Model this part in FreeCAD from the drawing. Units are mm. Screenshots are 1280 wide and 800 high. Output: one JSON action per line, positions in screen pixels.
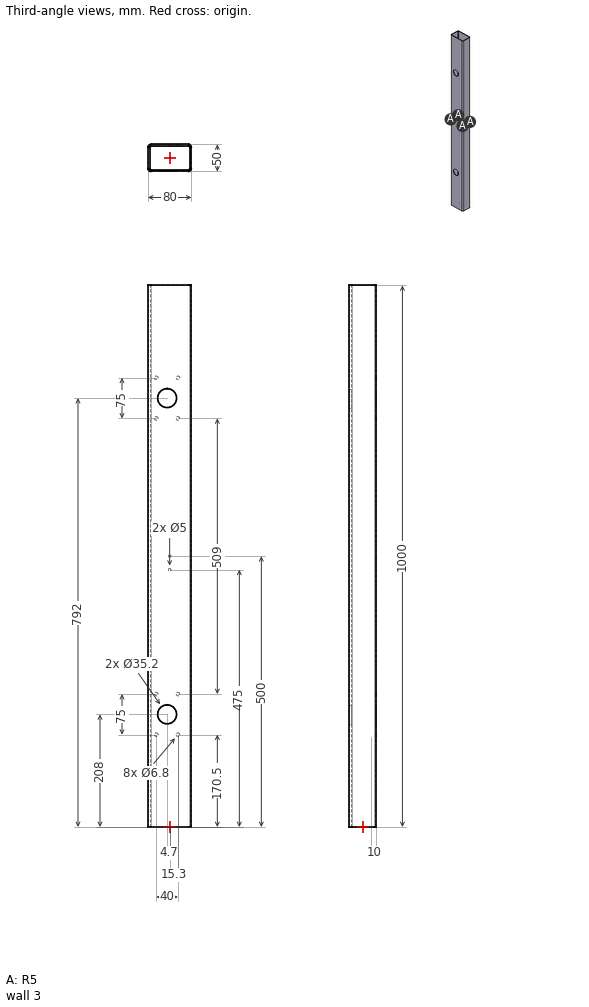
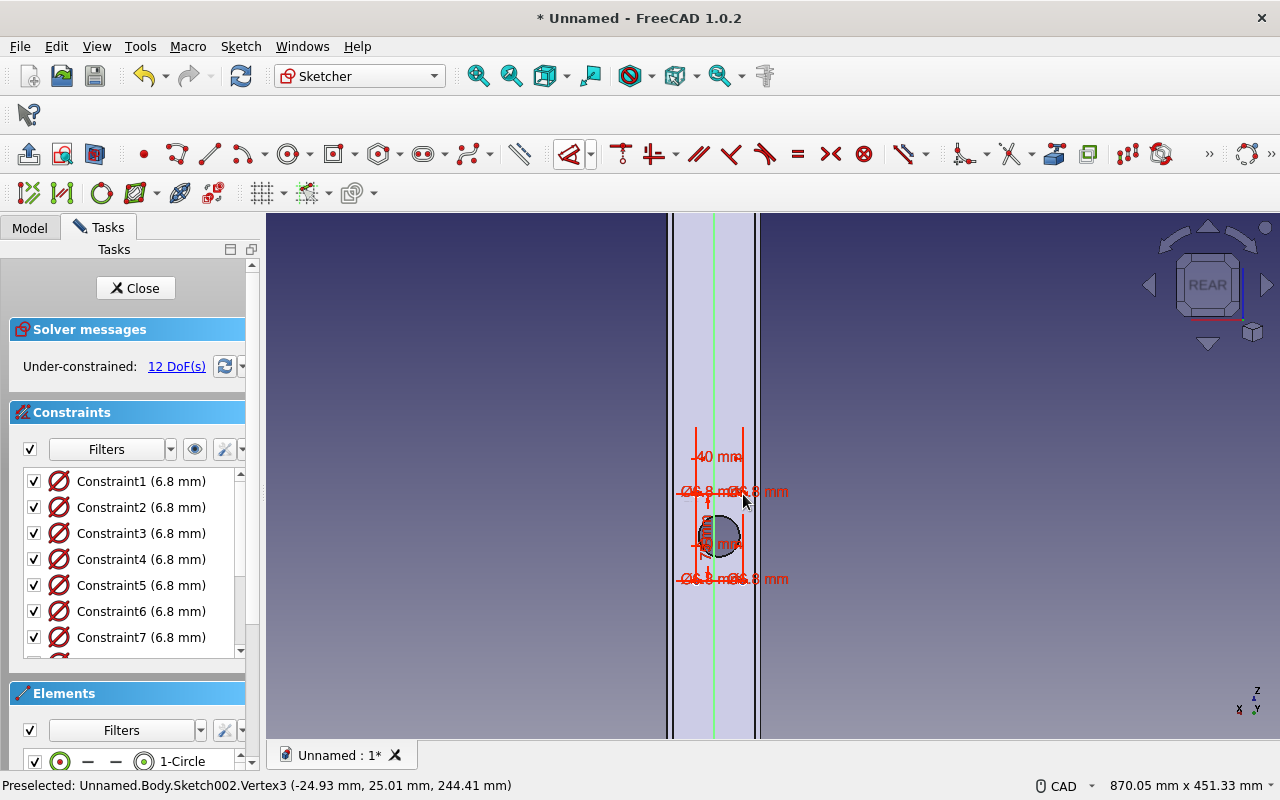
{"action": "left_click", "coordinate": [696, 494]}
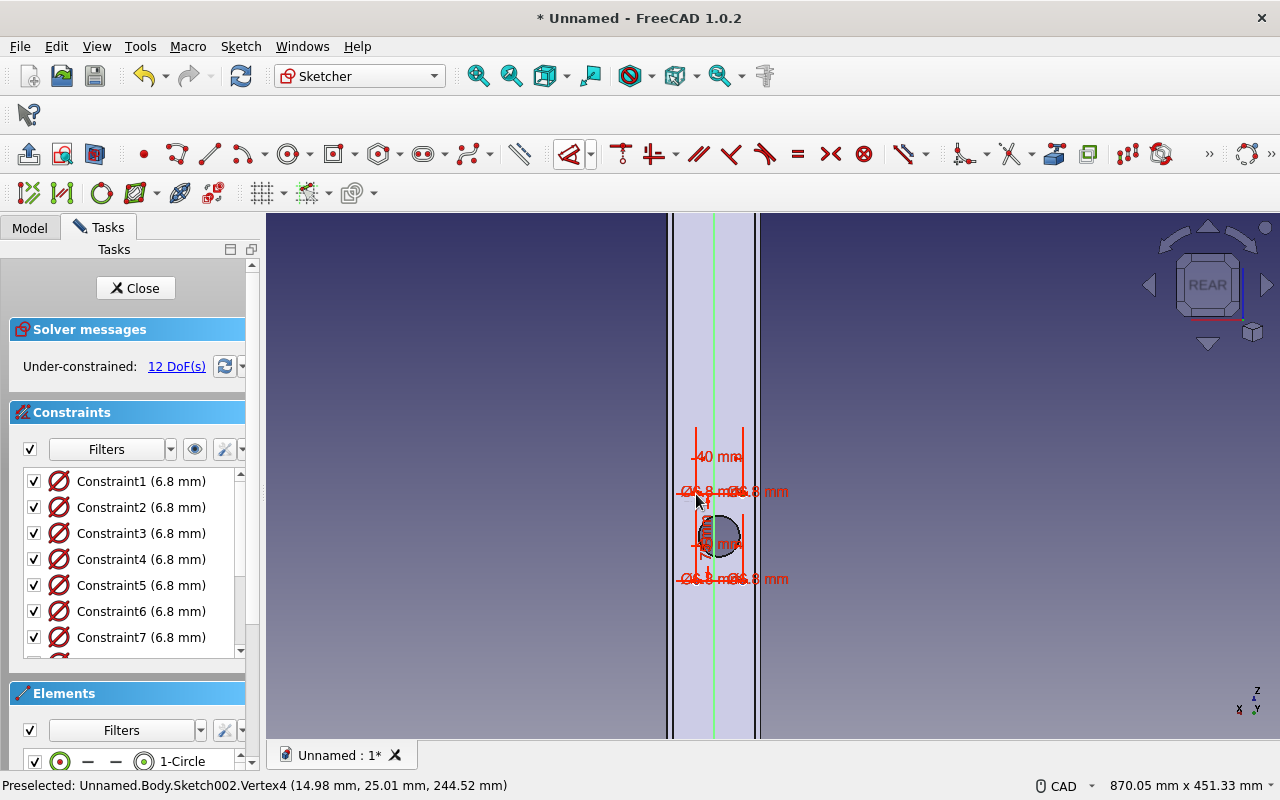
{"action": "key", "text": "l"}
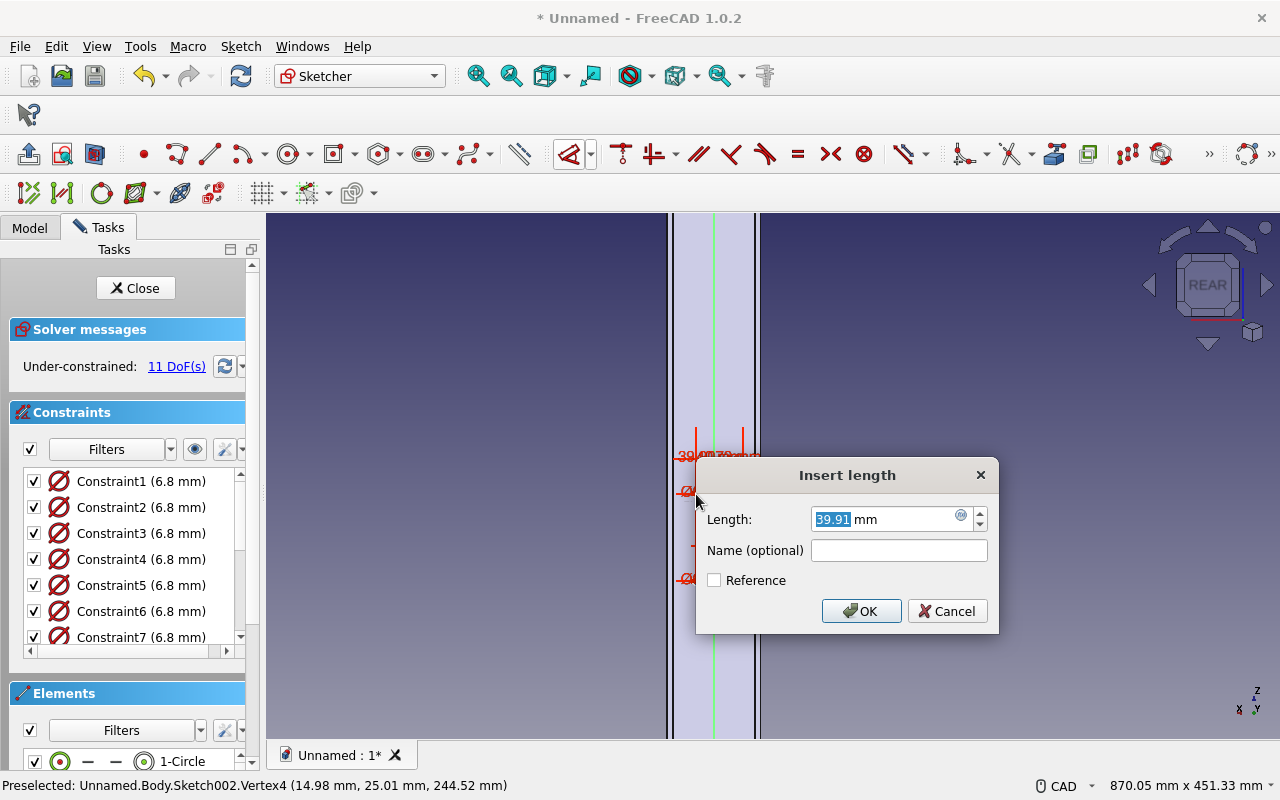
{"action": "type", "text": "40"}
{"action": "key", "text": "Return"}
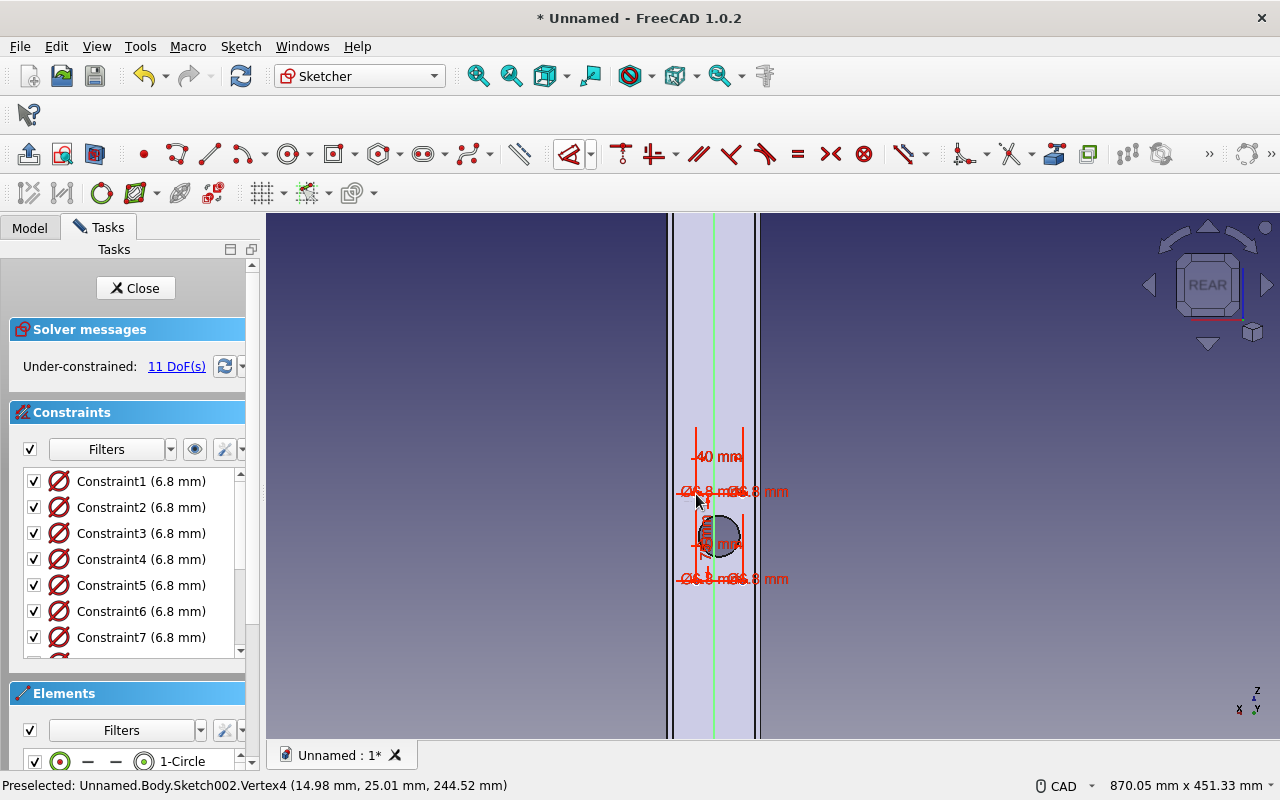
{"action": "left_click", "coordinate": [696, 581]}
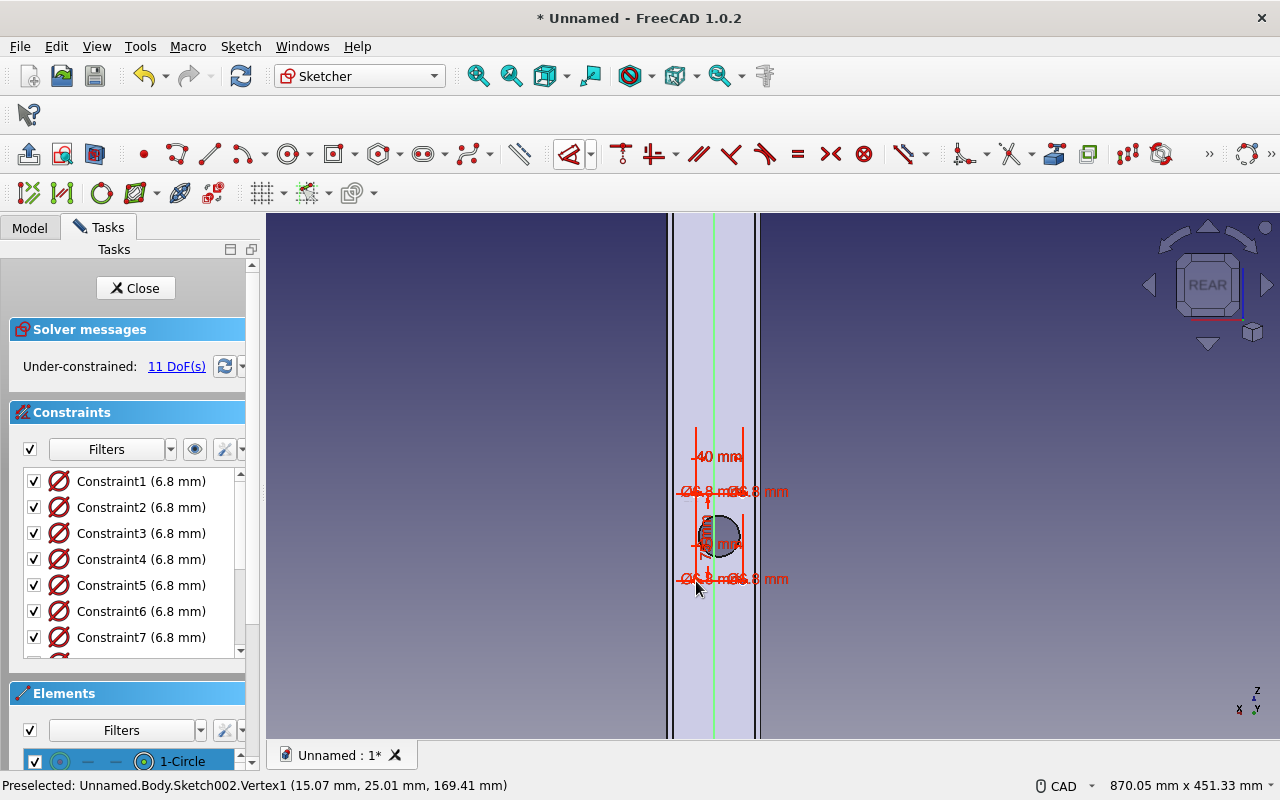
{"action": "left_click", "coordinate": [696, 494]}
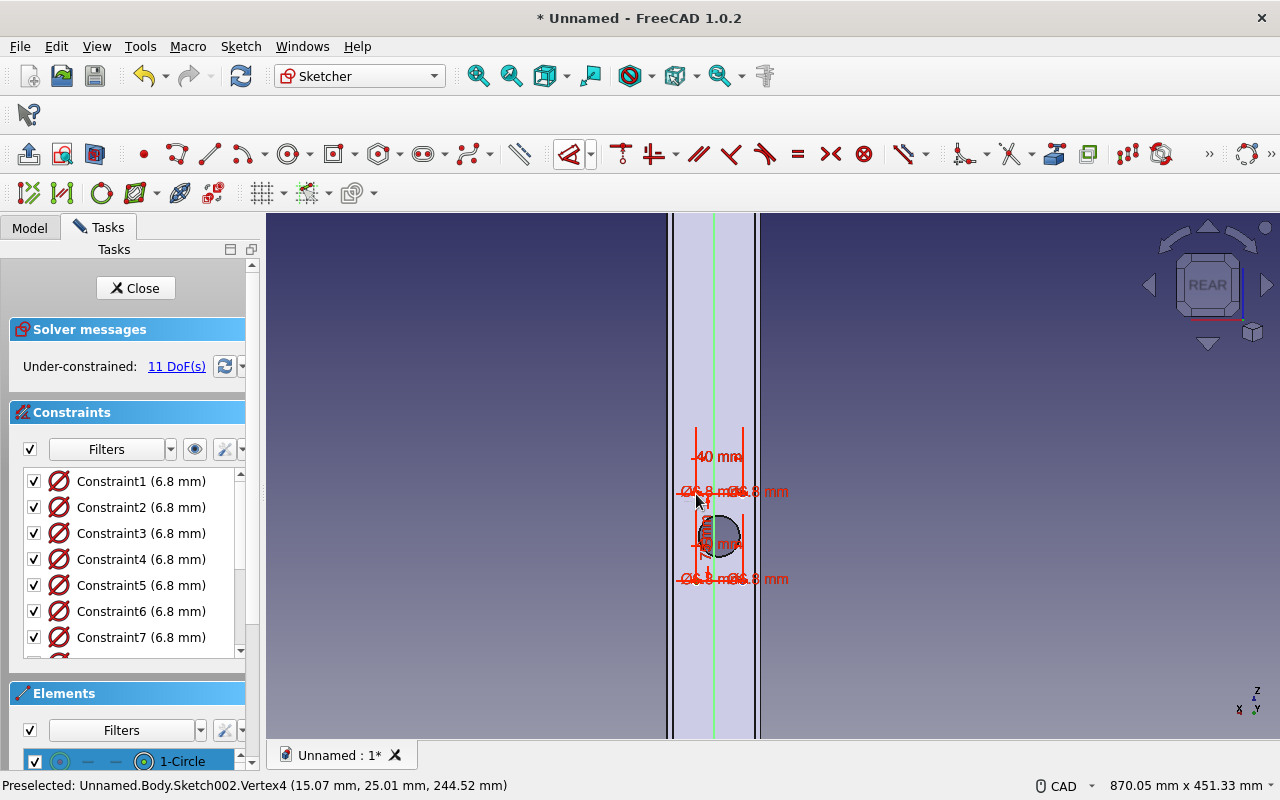
{"action": "left_click", "coordinate": [590, 154]}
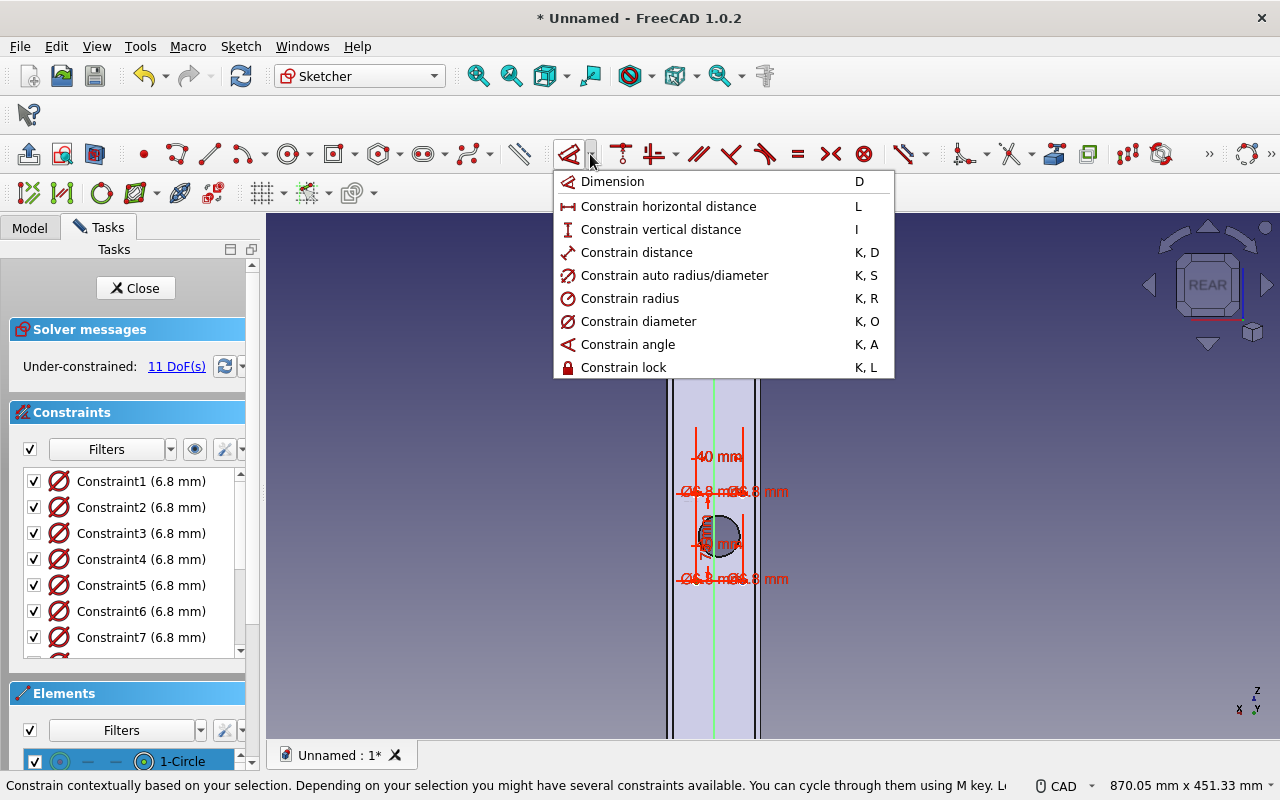
{"action": "left_click", "coordinate": [724, 230]}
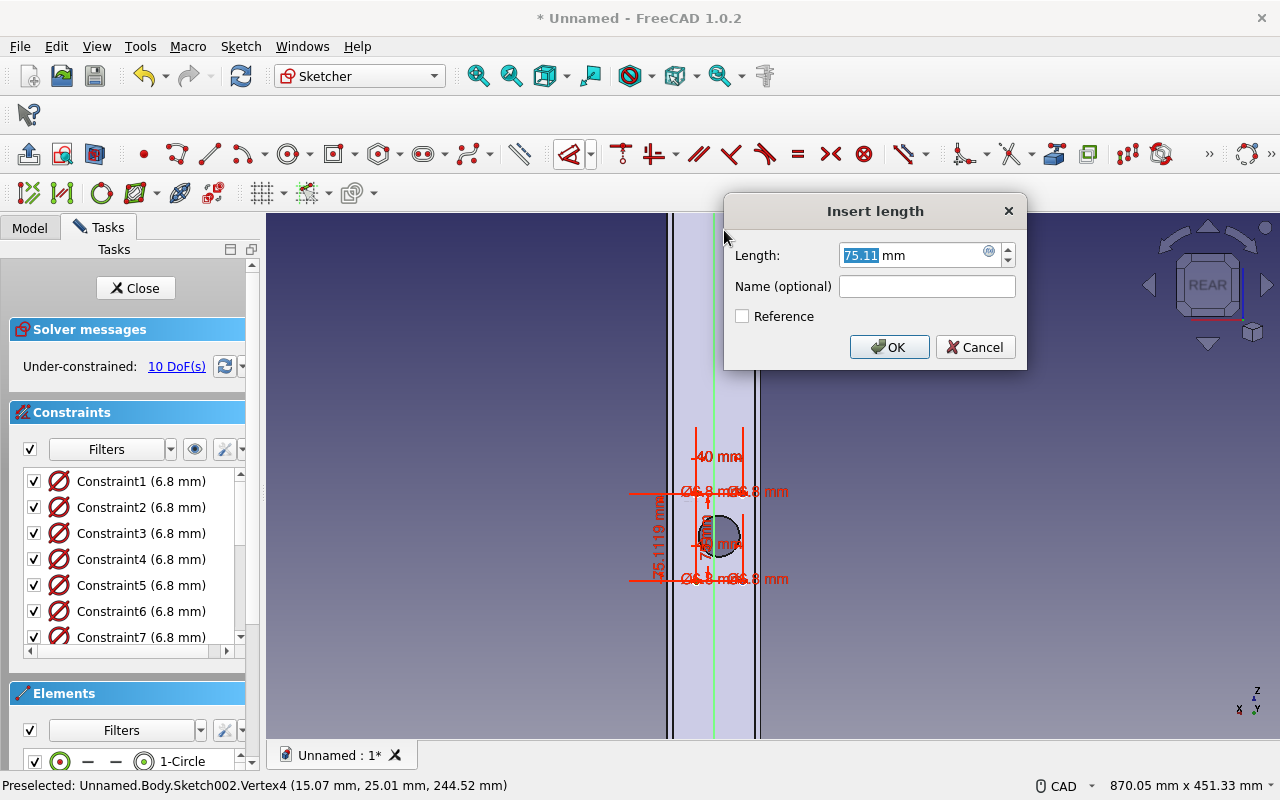
{"action": "type", "text": "75"}
{"action": "key", "text": "Return"}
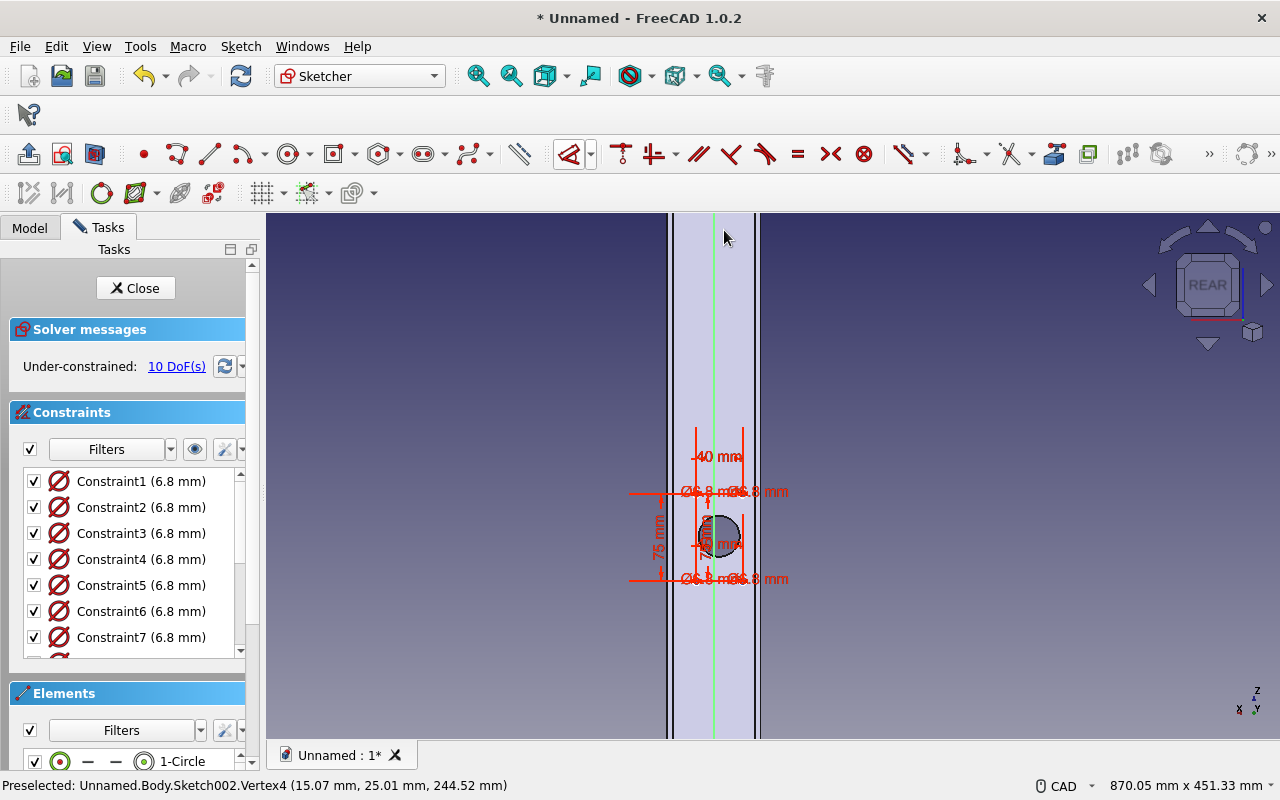
{"action": "left_click", "coordinate": [743, 494]}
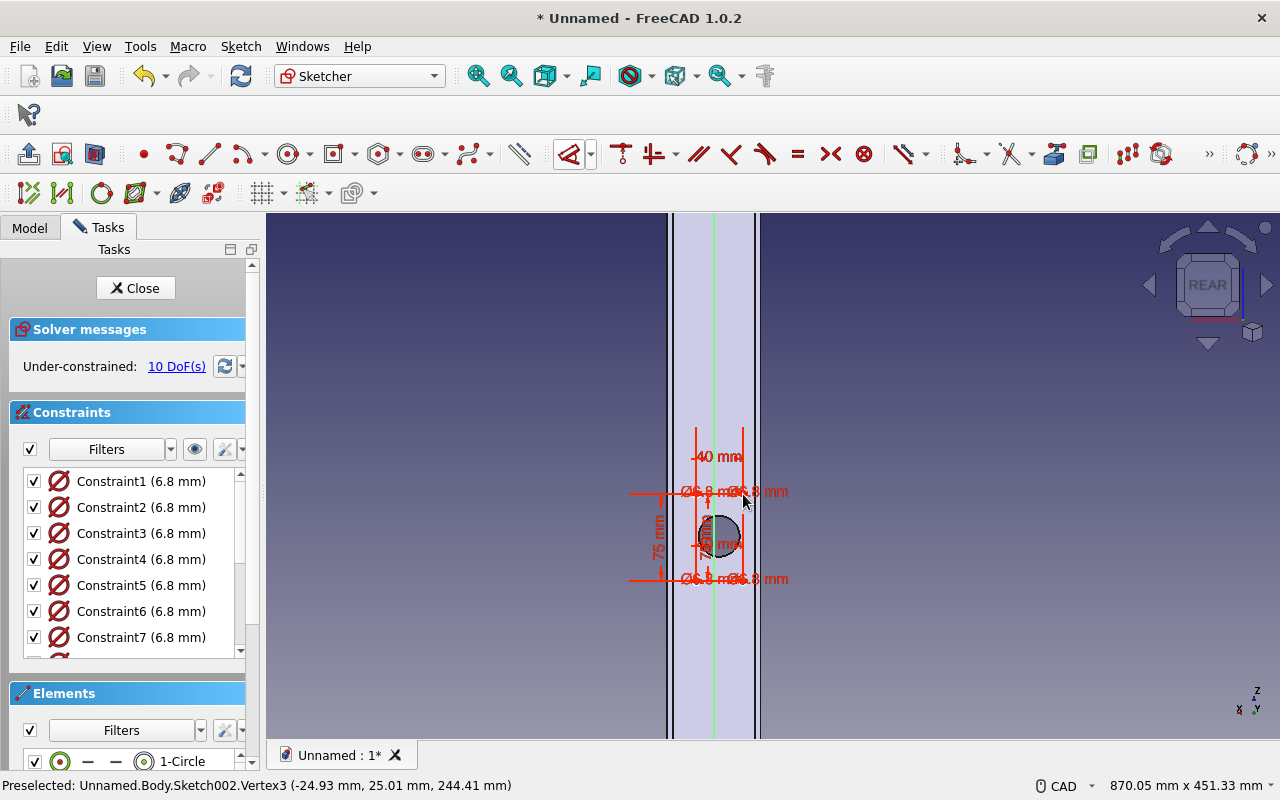
{"action": "scroll", "coordinate": [696, 582], "scroll_direction": "down", "scroll_amount": 5}